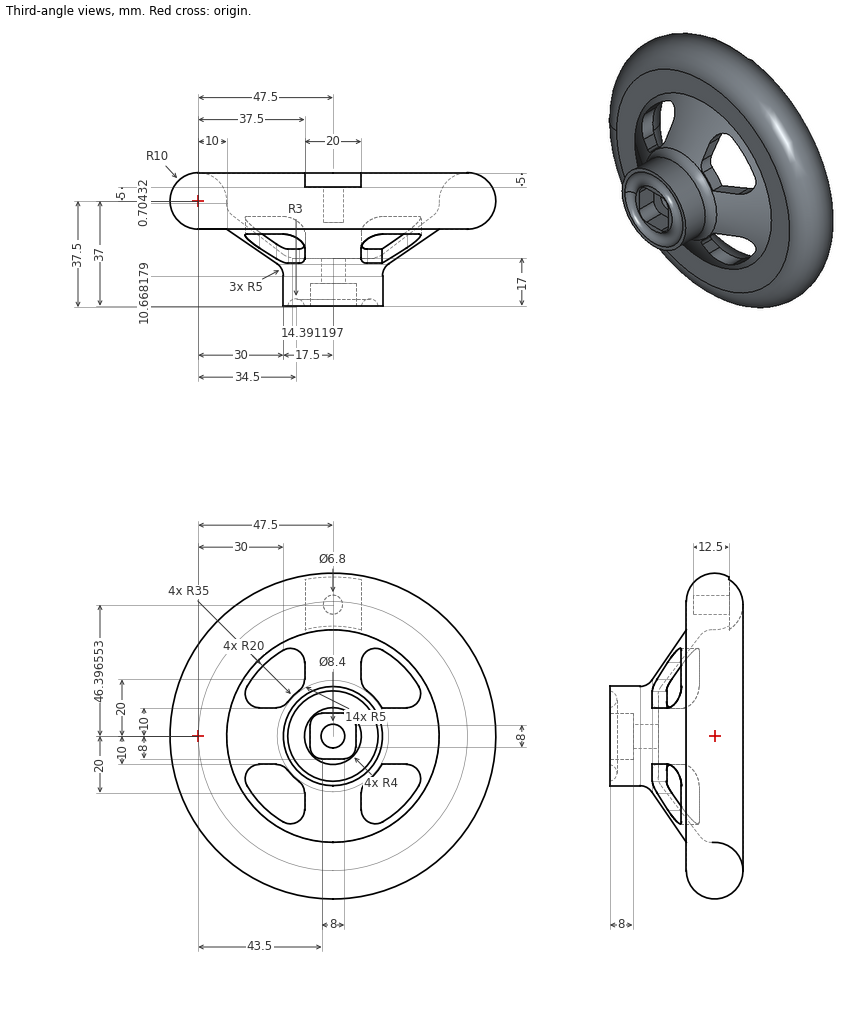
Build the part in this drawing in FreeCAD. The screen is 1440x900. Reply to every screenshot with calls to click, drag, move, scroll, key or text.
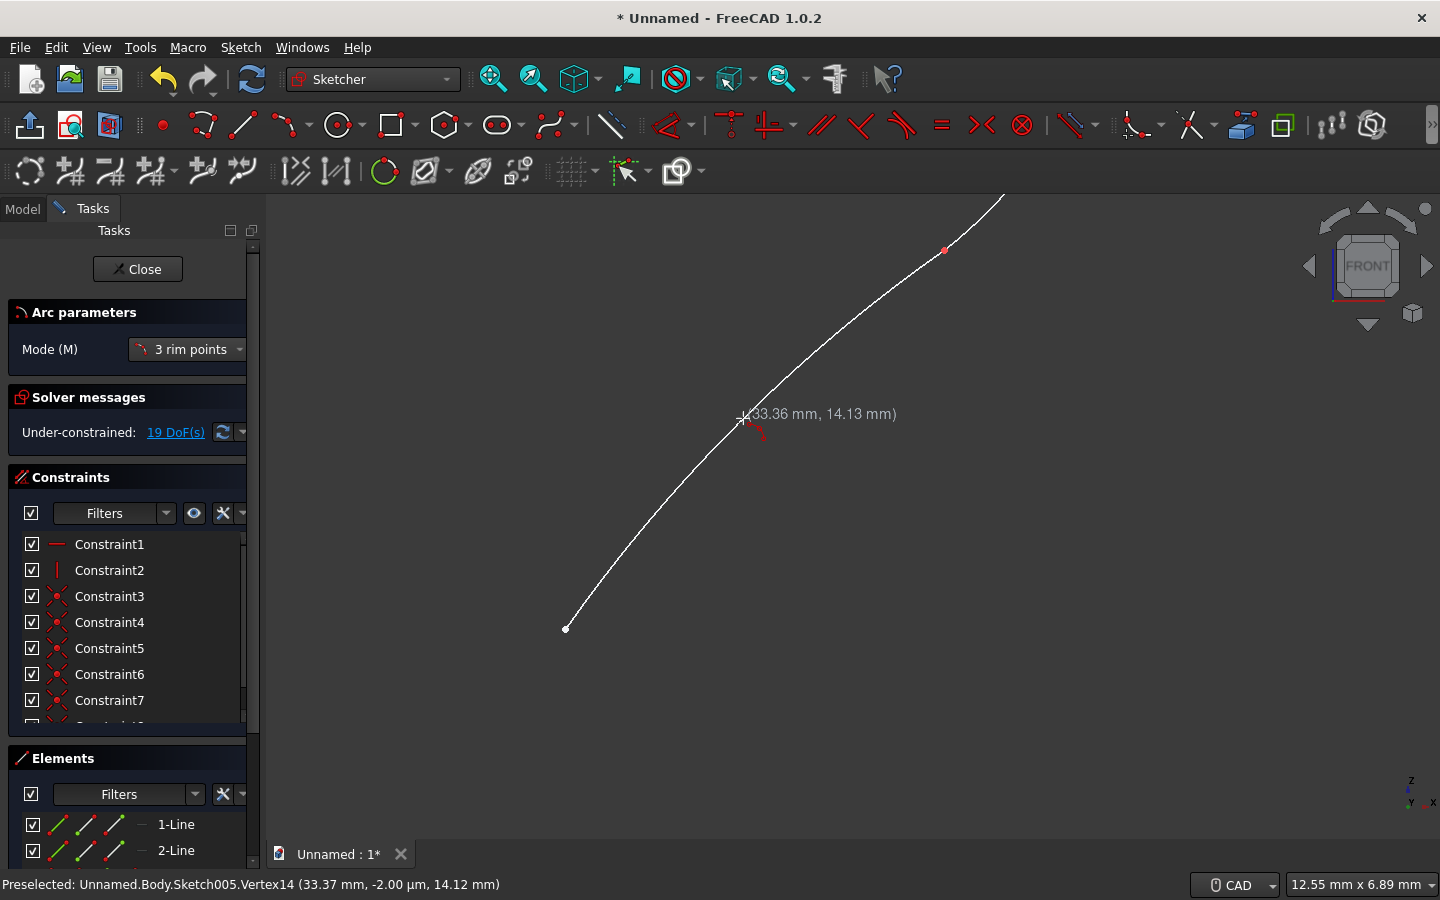
scroll(746, 418, down, 13)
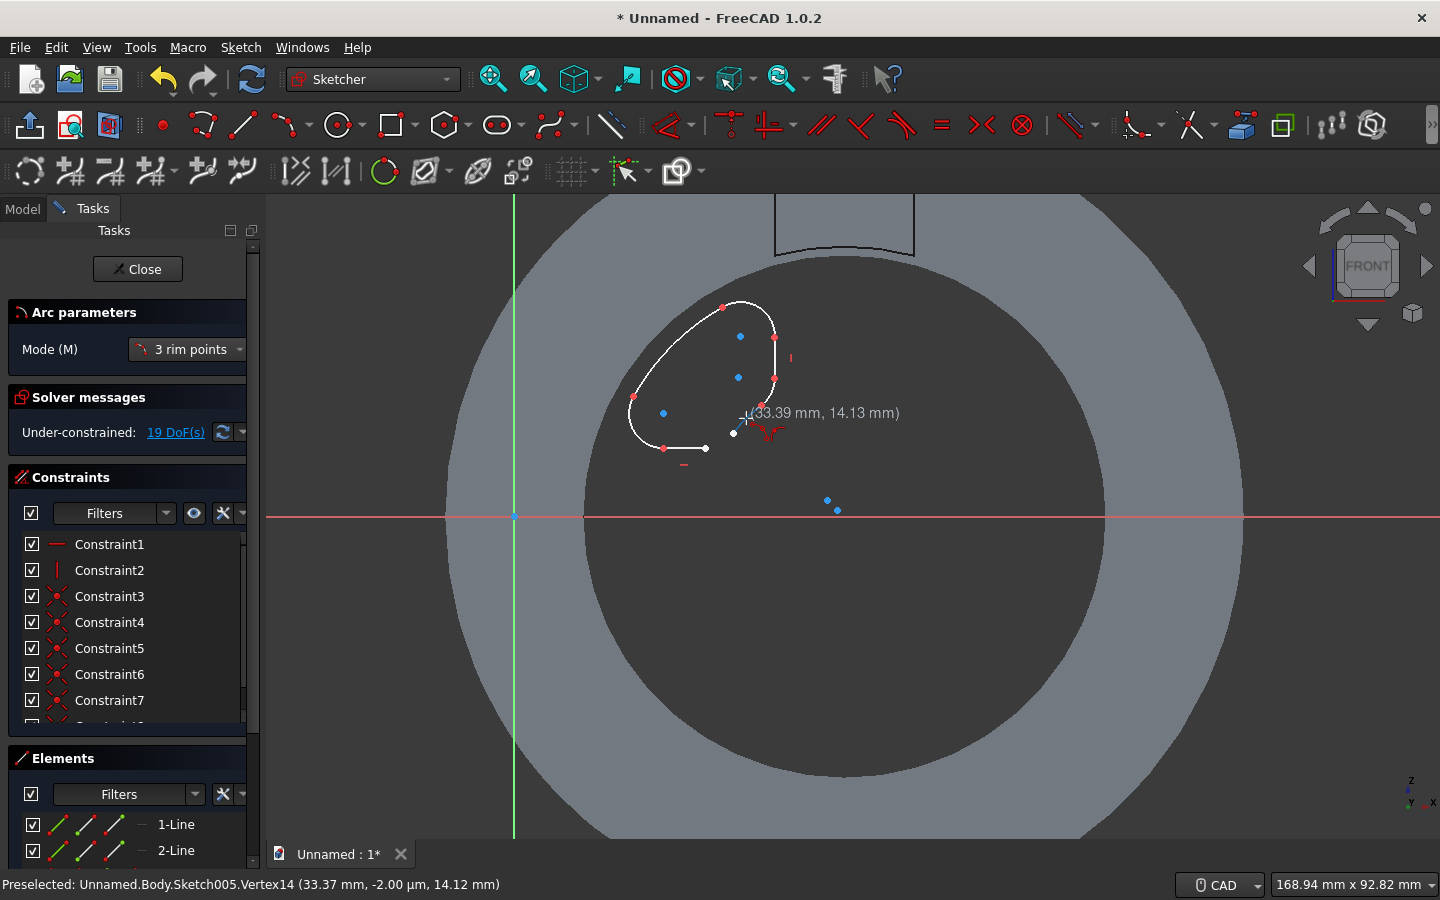
click(733, 434)
click(706, 448)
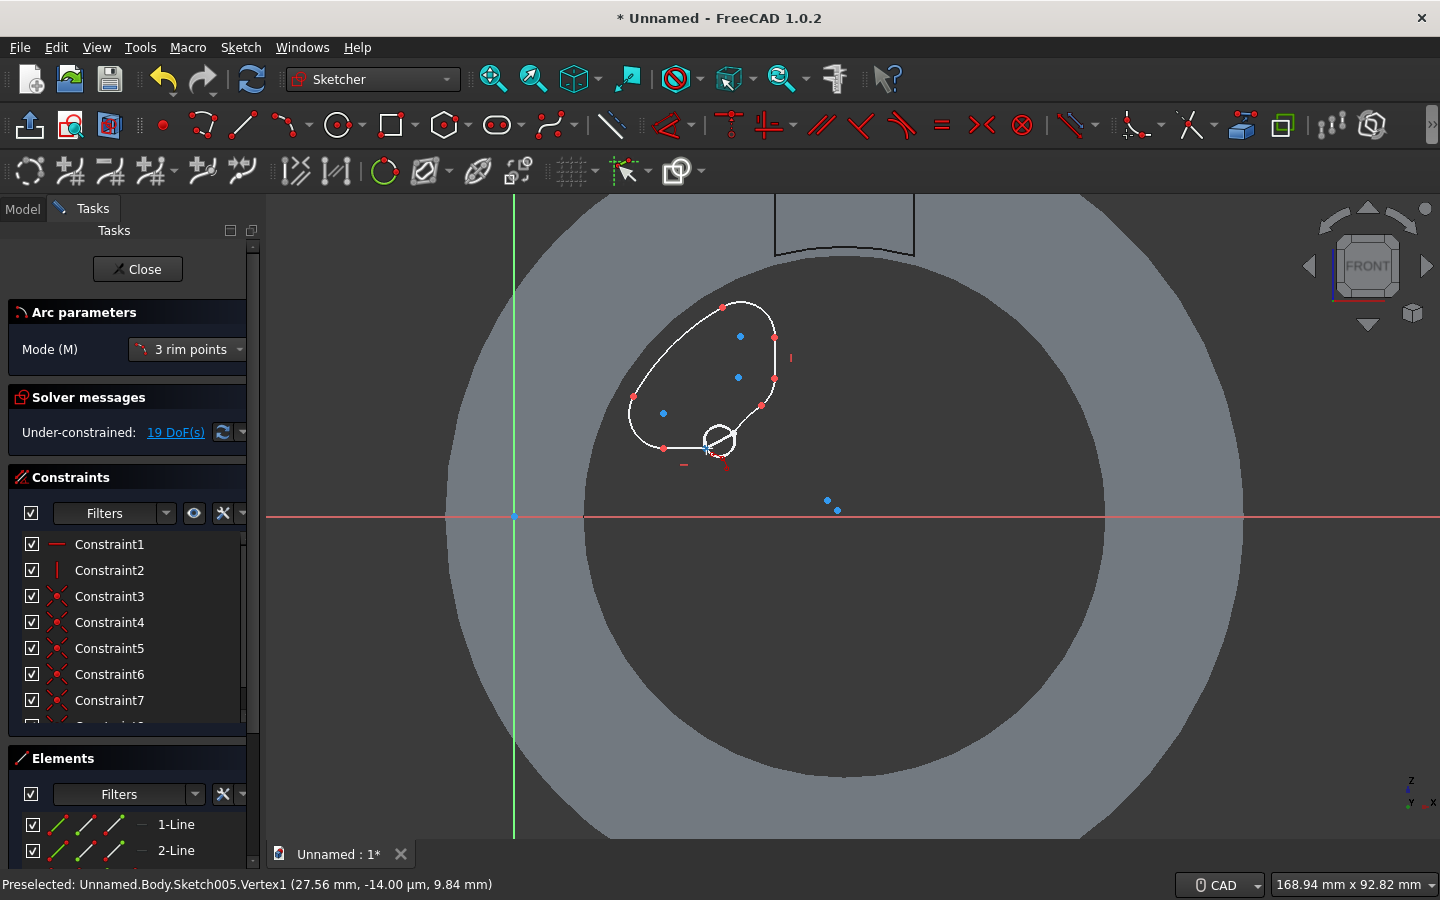
scroll(721, 443, up, 8)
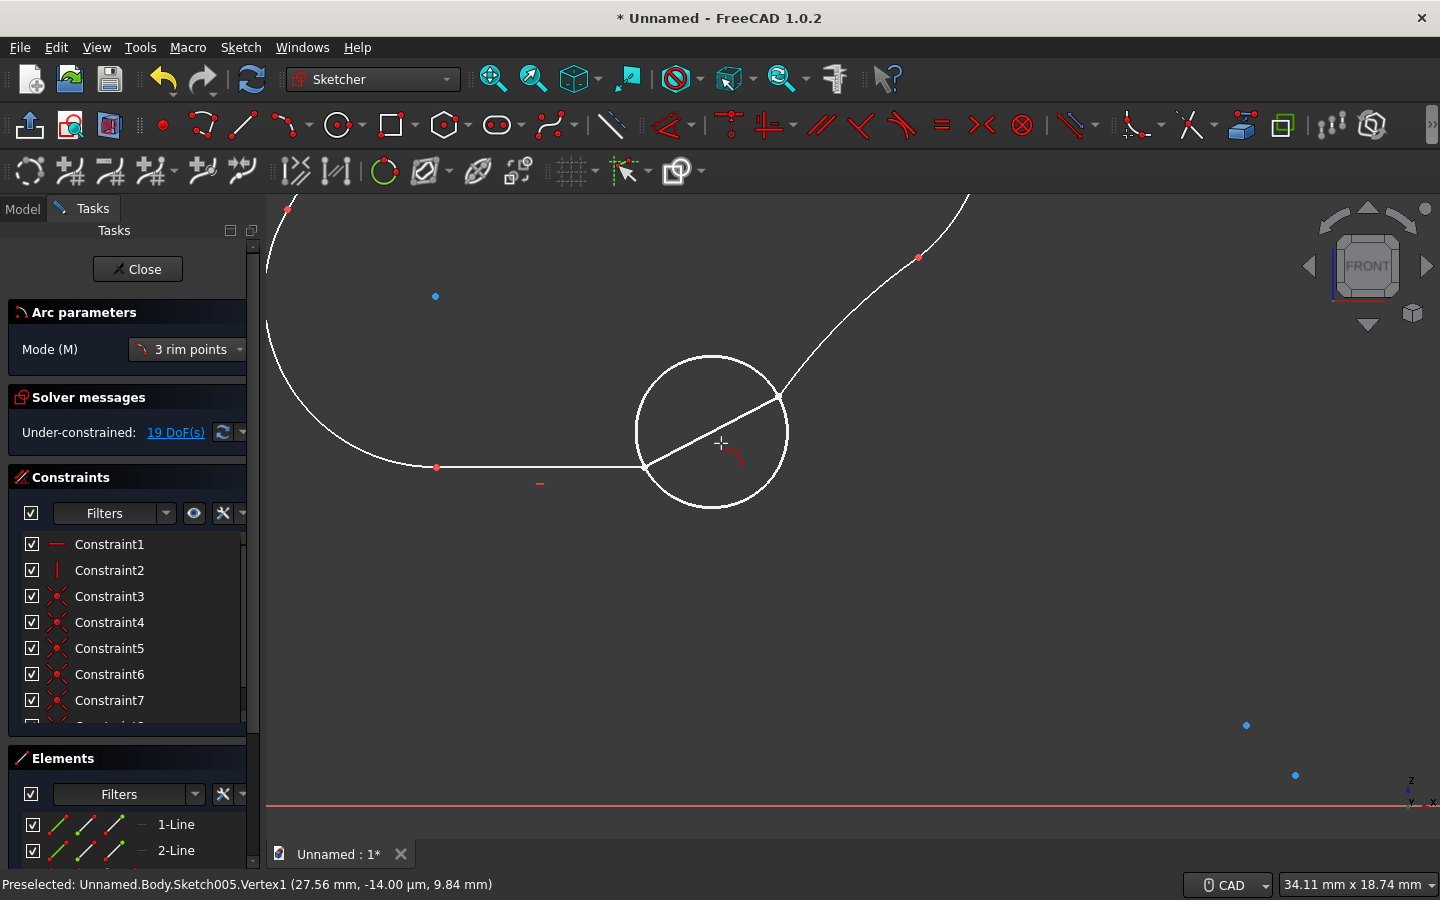
click(719, 443)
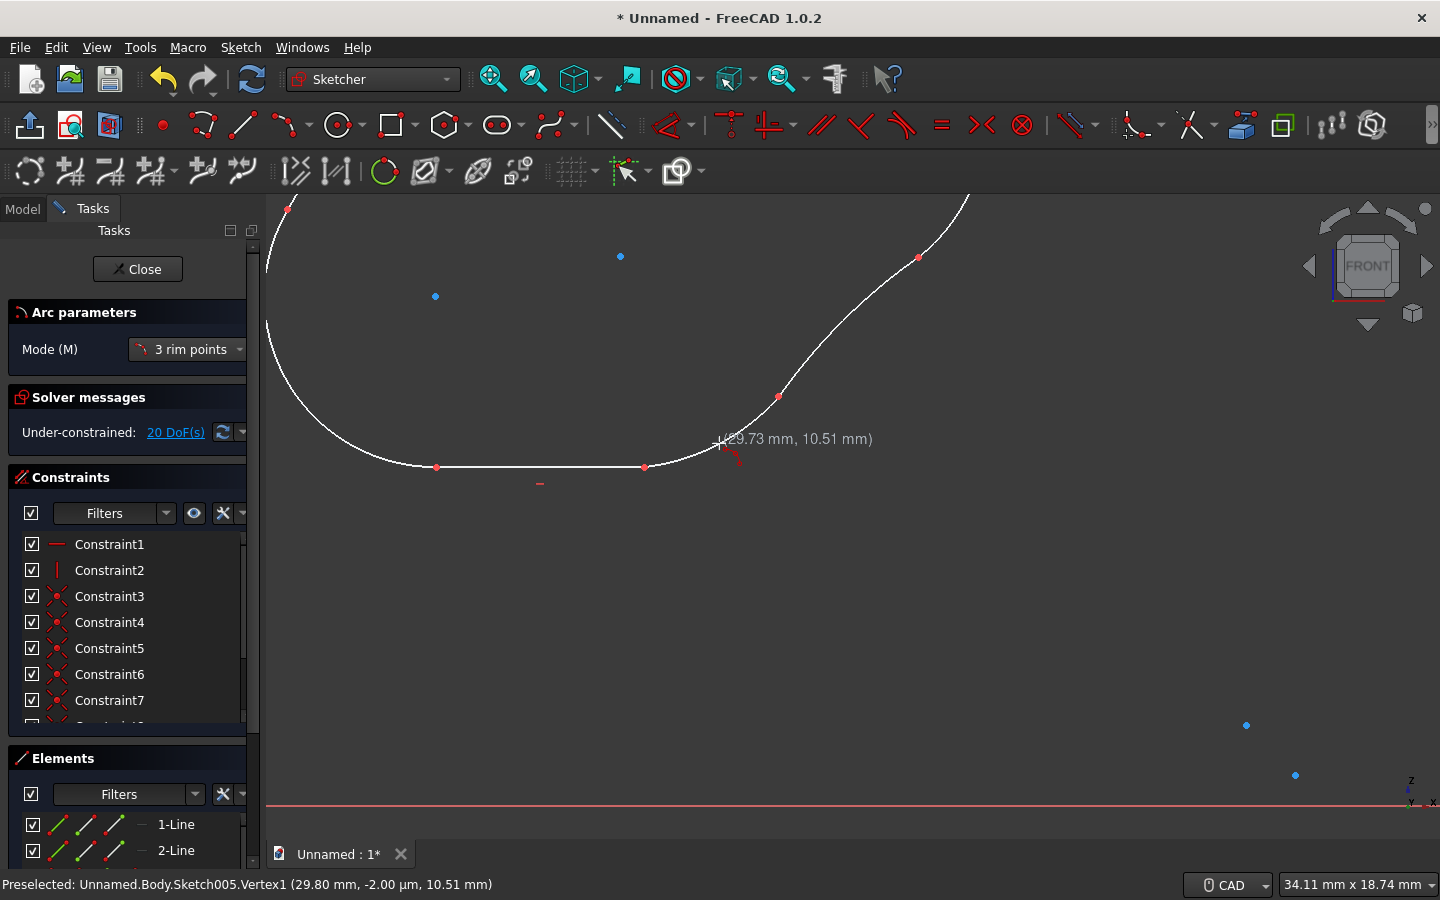
click(244, 126)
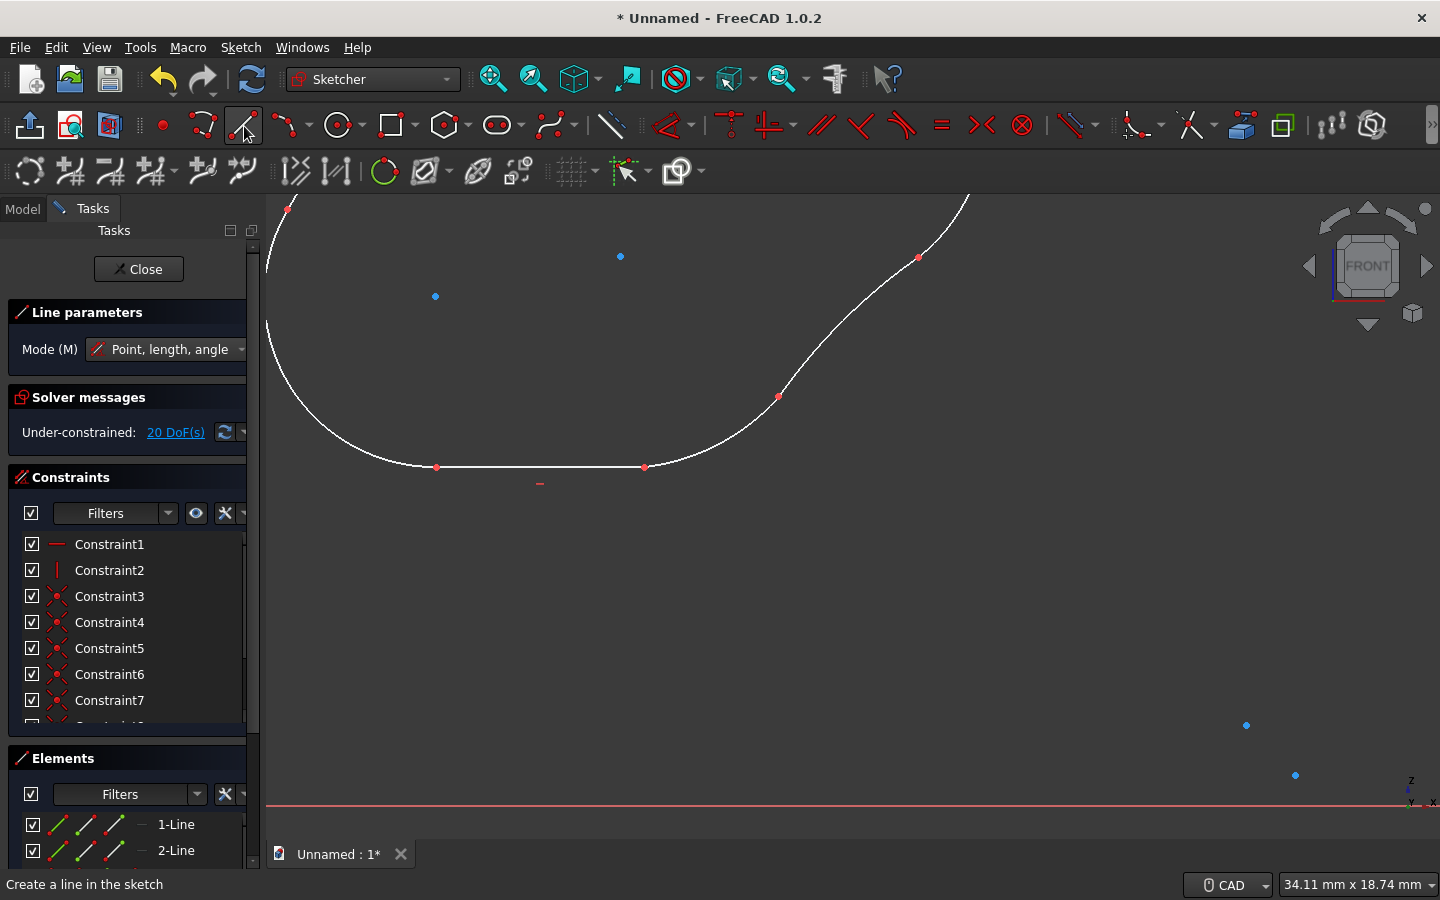
scroll(721, 443, down, 8)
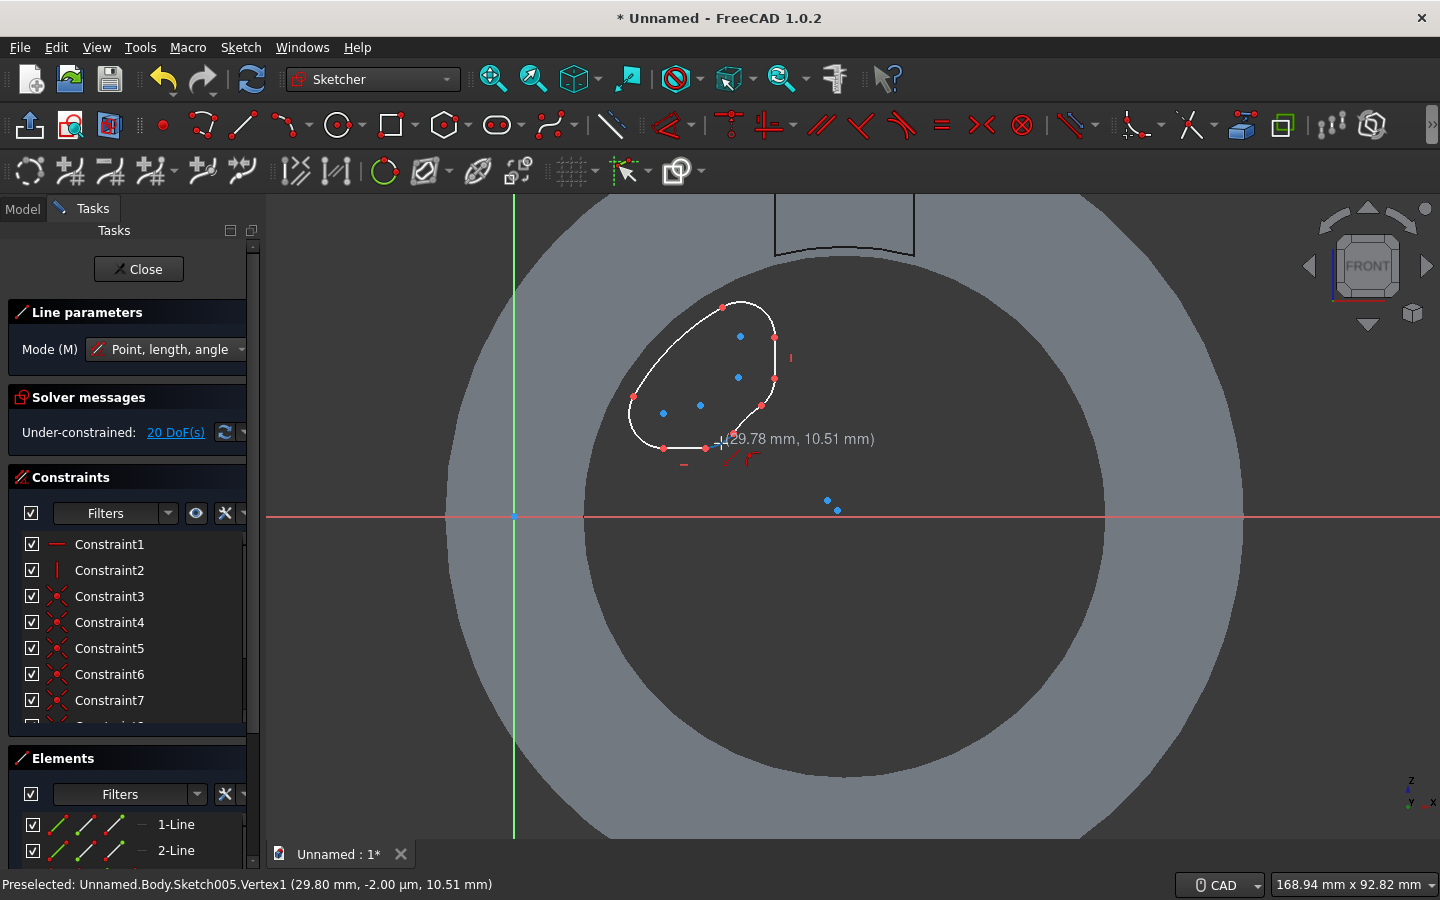
click(664, 586)
click(705, 586)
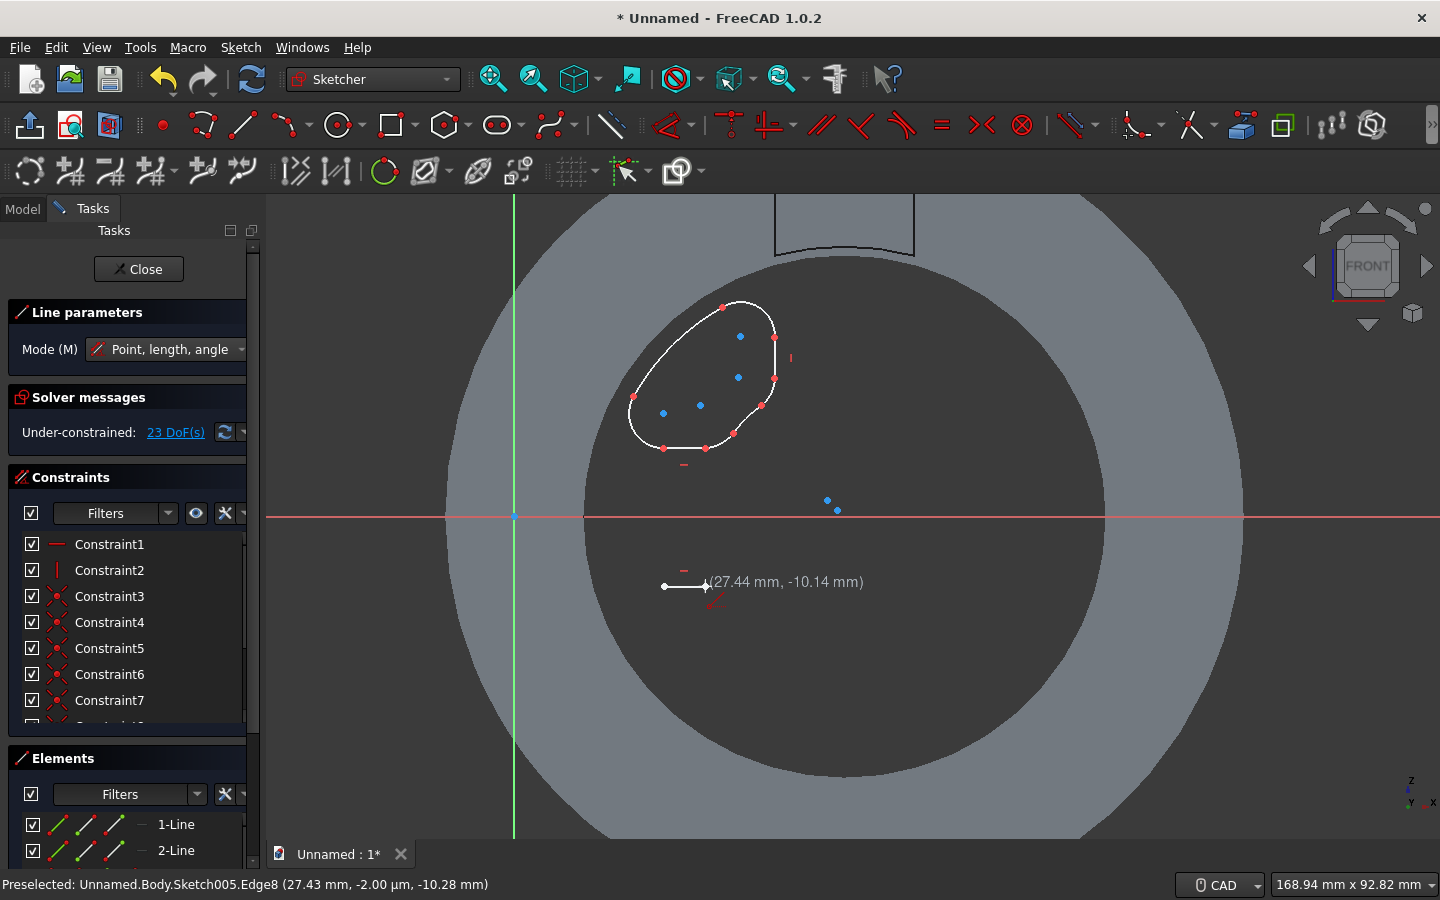
click(775, 656)
click(775, 697)